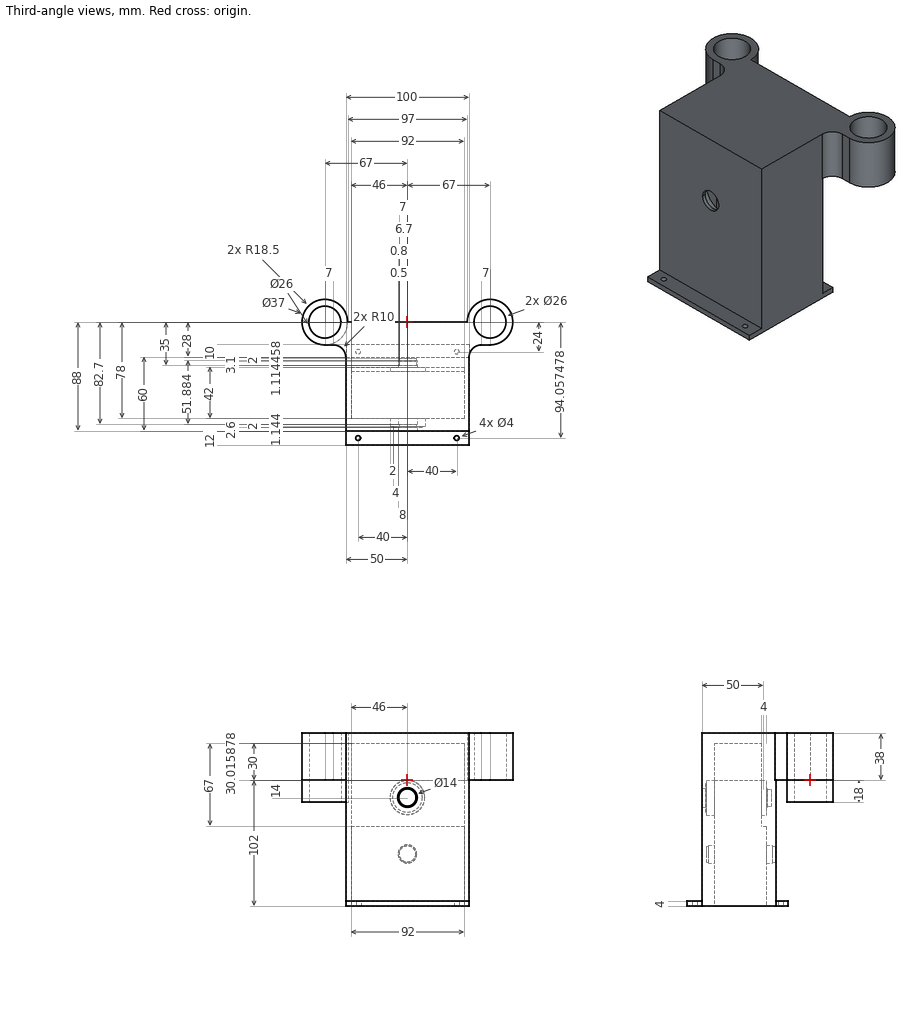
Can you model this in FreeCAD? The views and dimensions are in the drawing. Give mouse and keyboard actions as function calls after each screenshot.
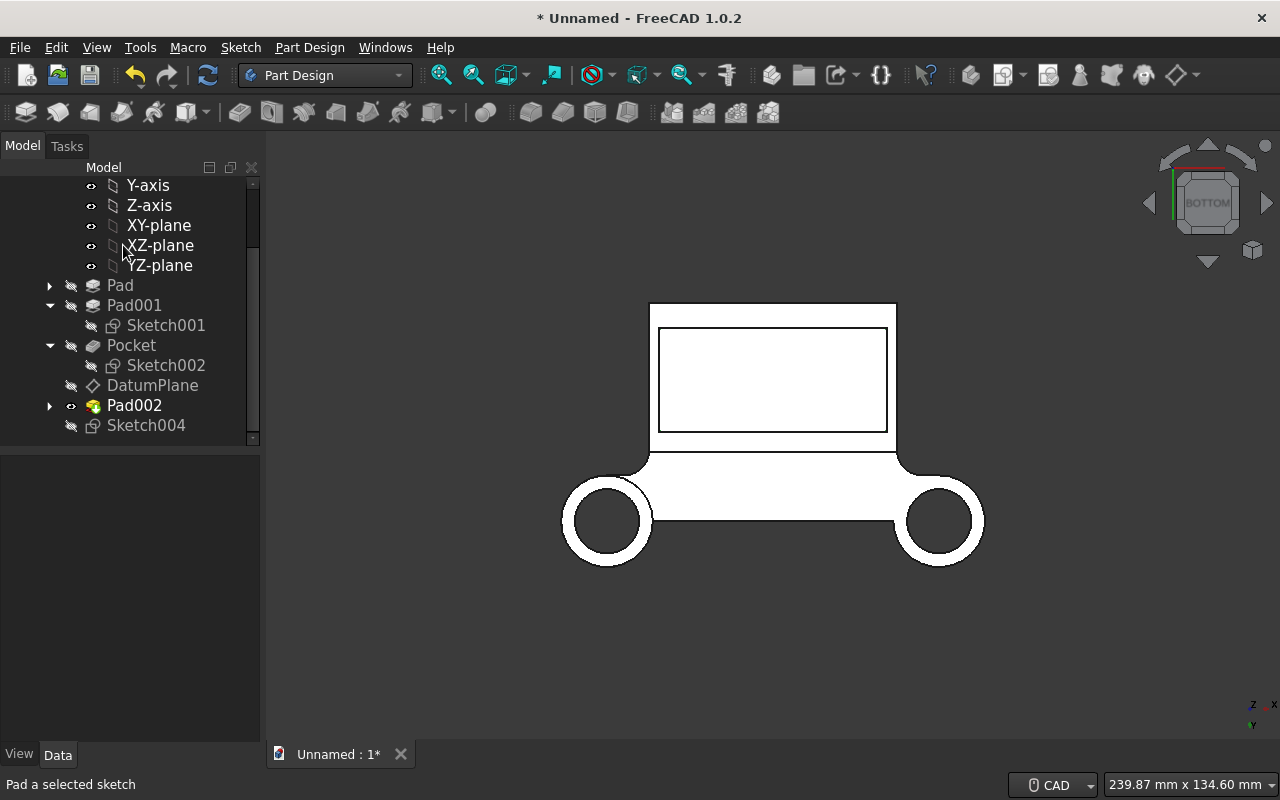
click(240, 112)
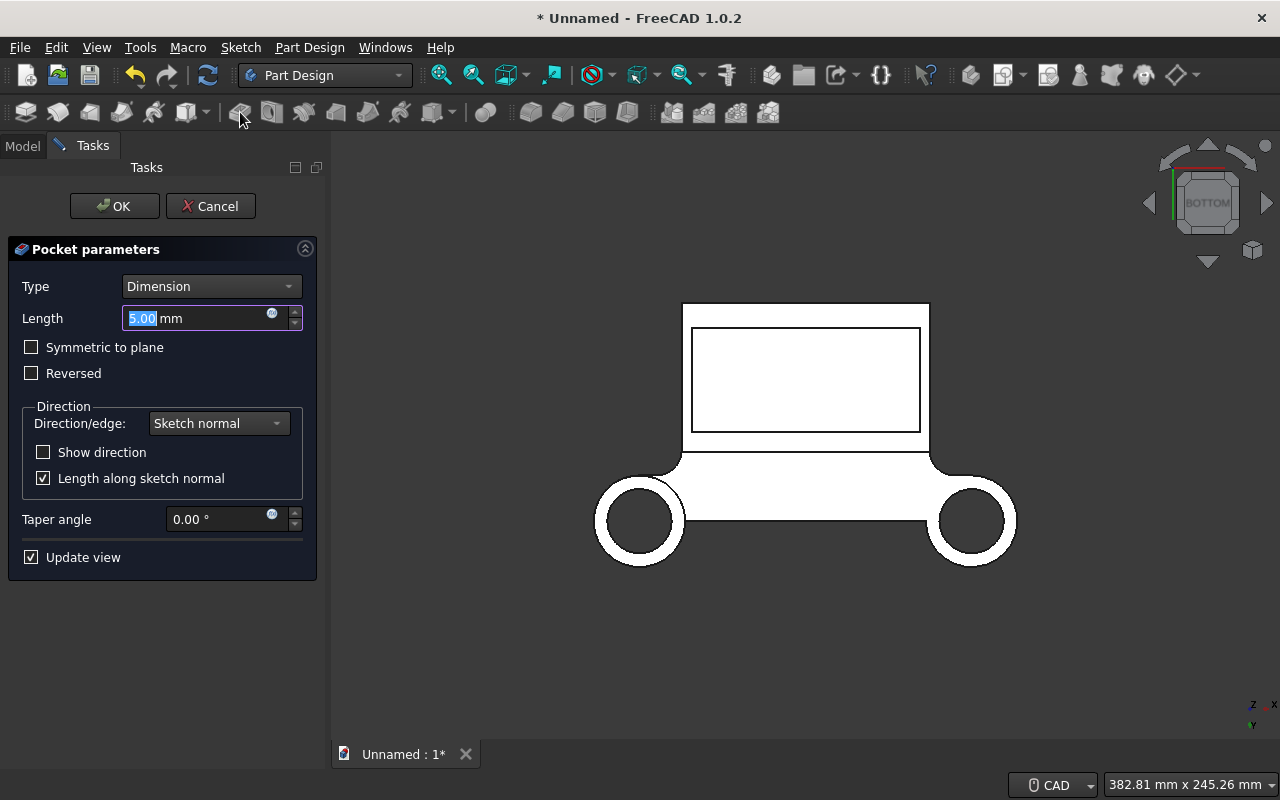
text(30)
key(Tab)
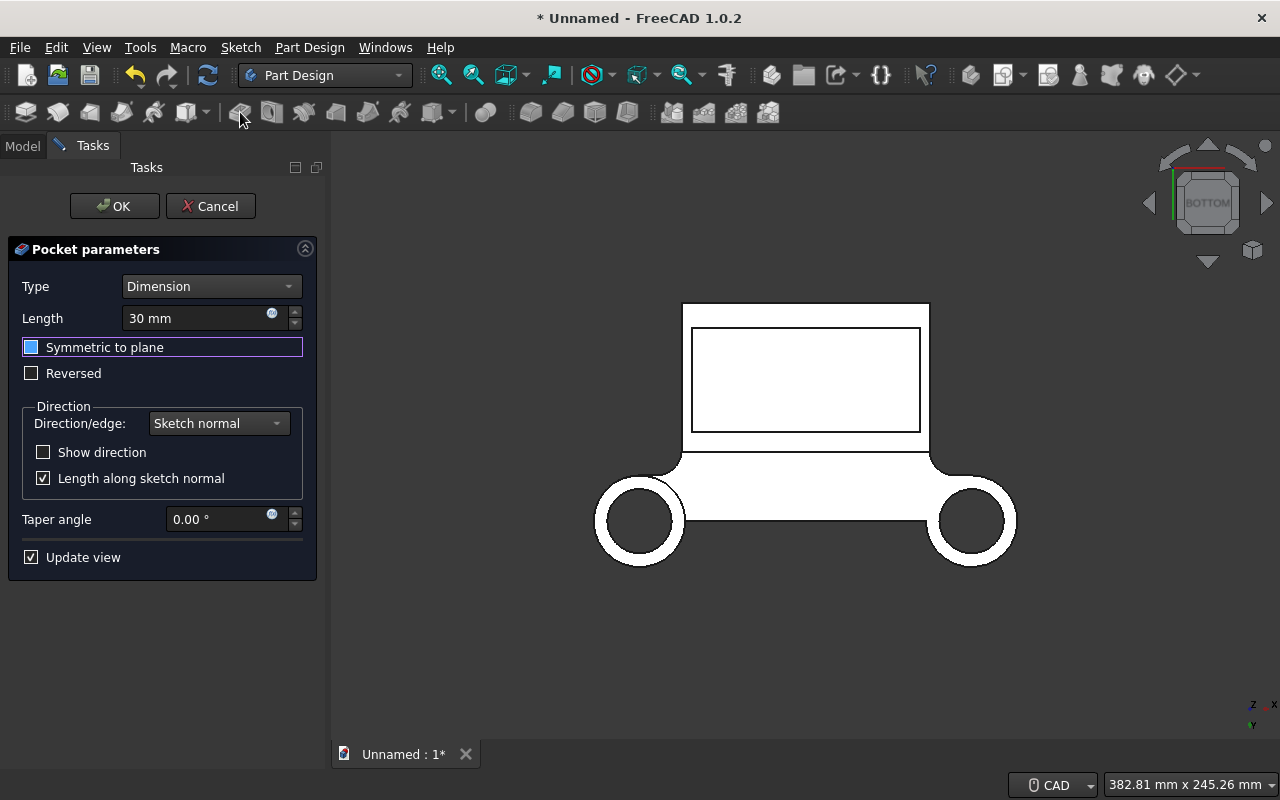
click(115, 206)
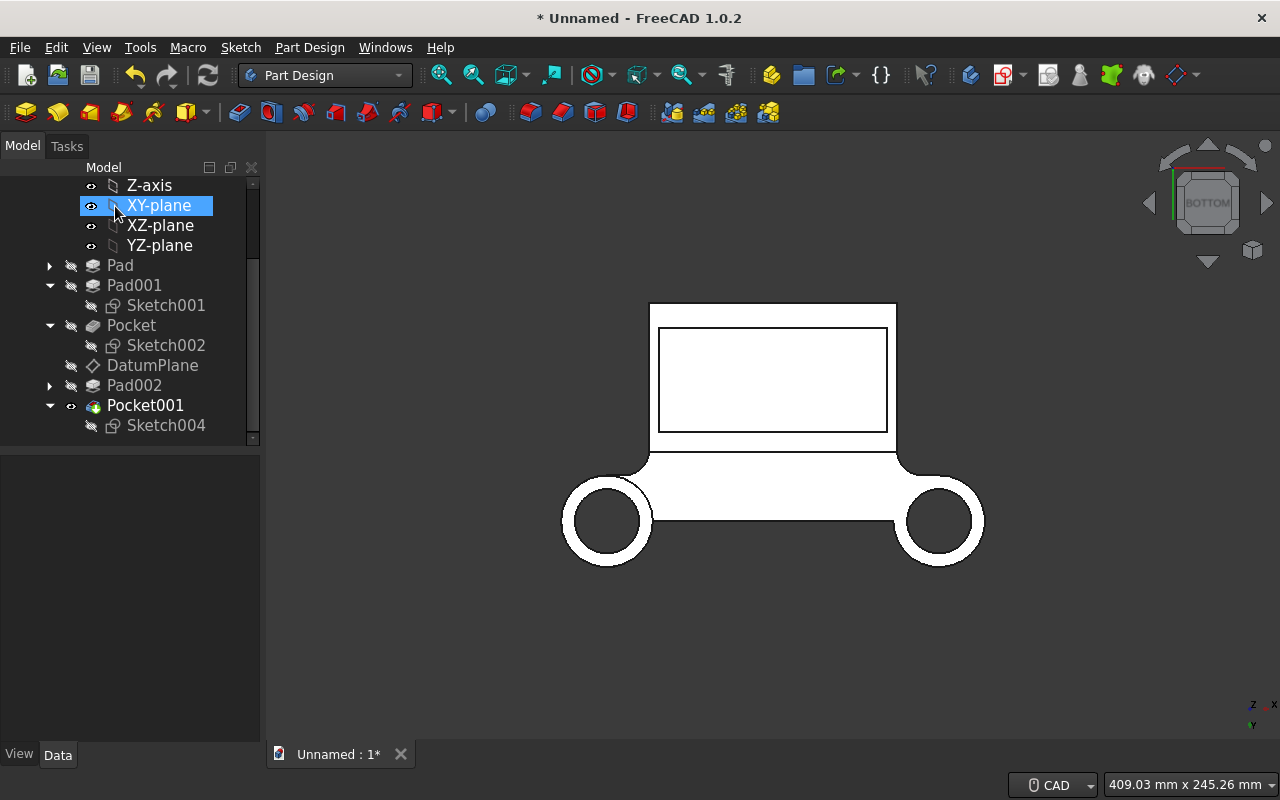
click(442, 76)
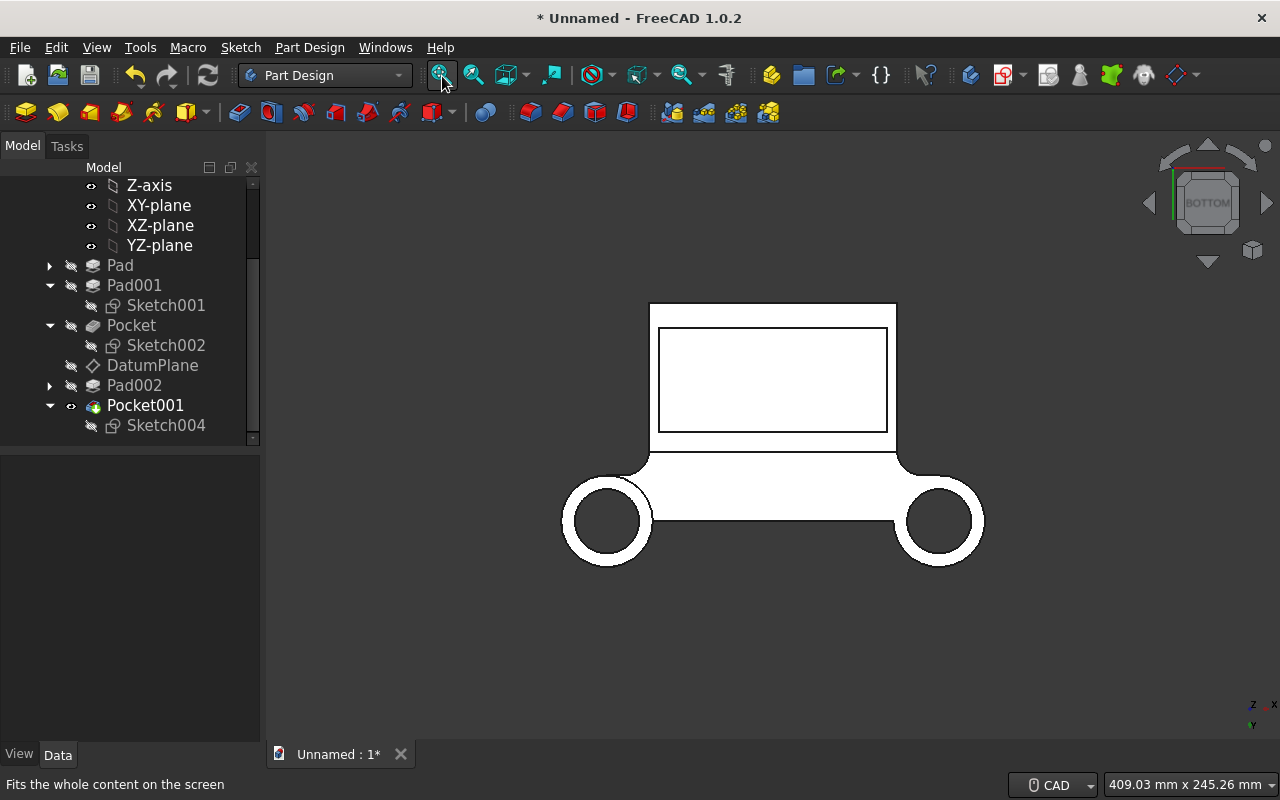
key(0)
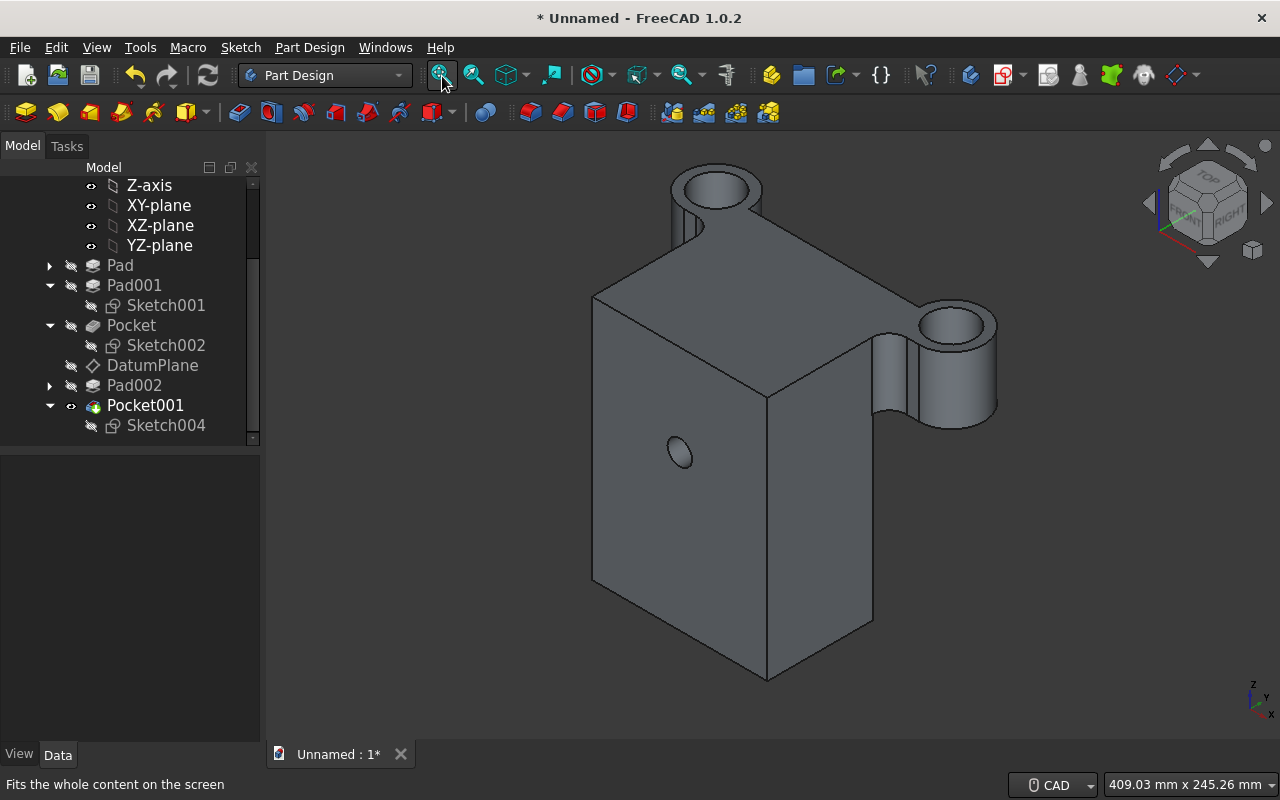
key(1)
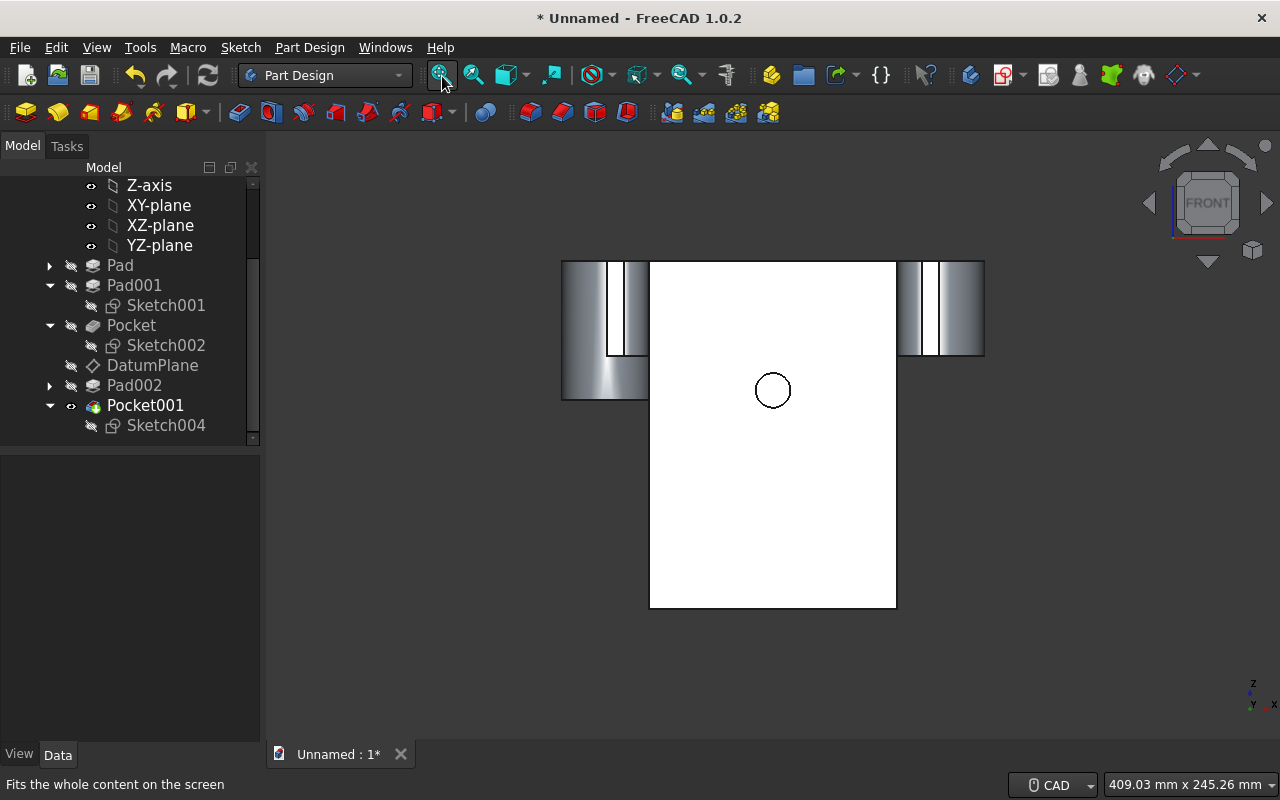
click(773, 397)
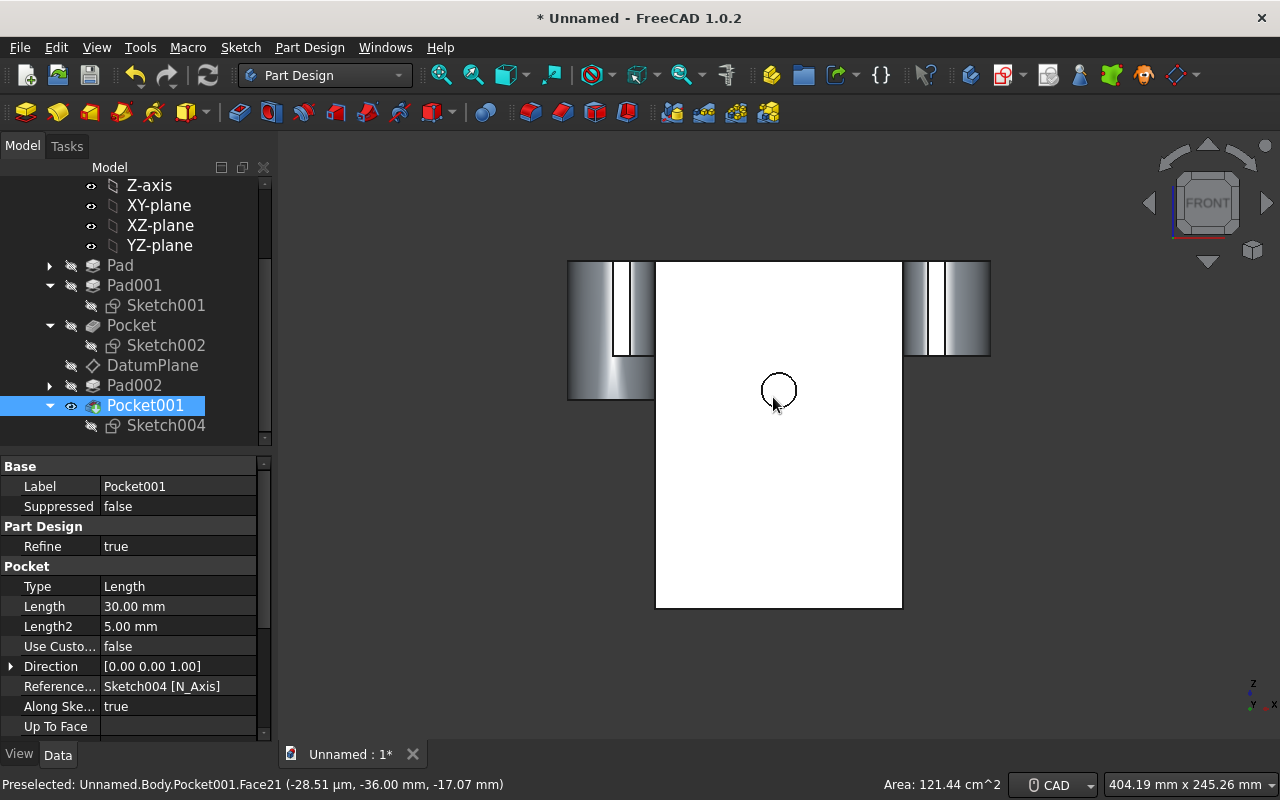
click(1004, 76)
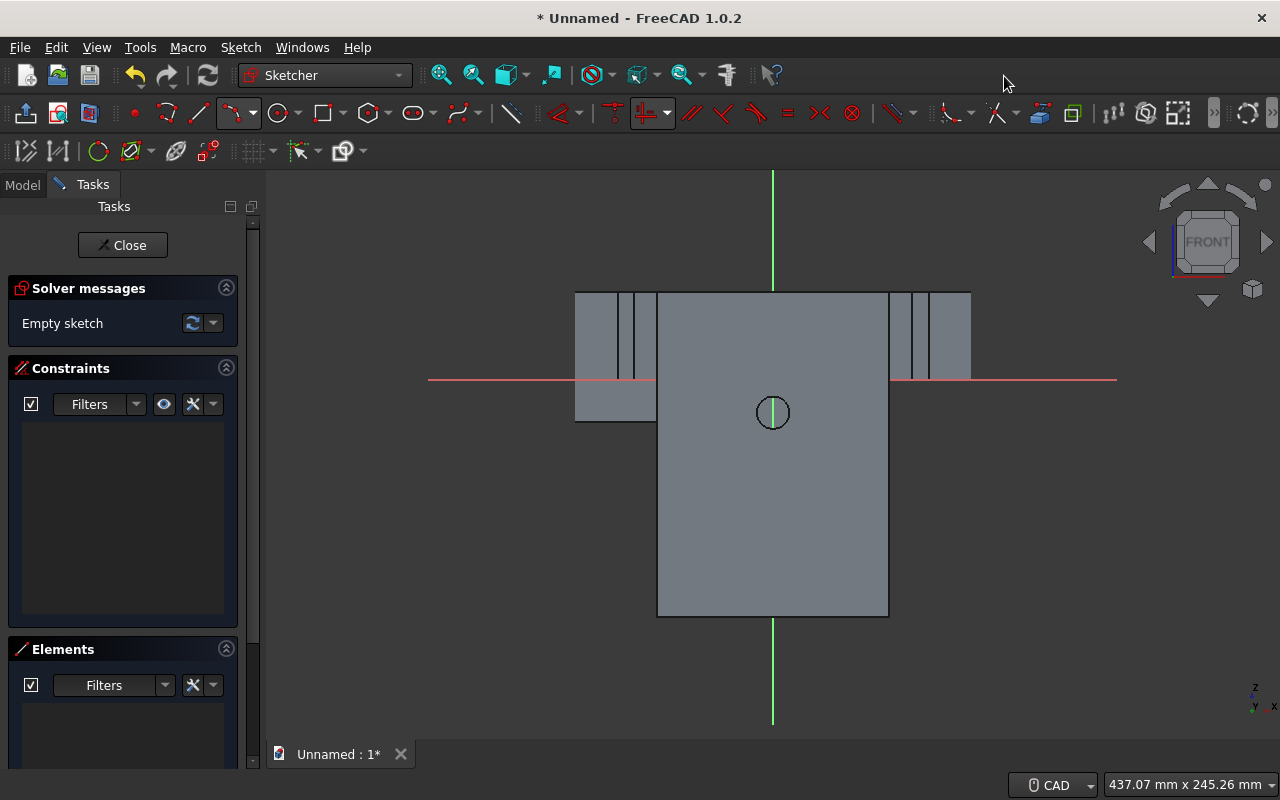
scroll(829, 334, up, 4)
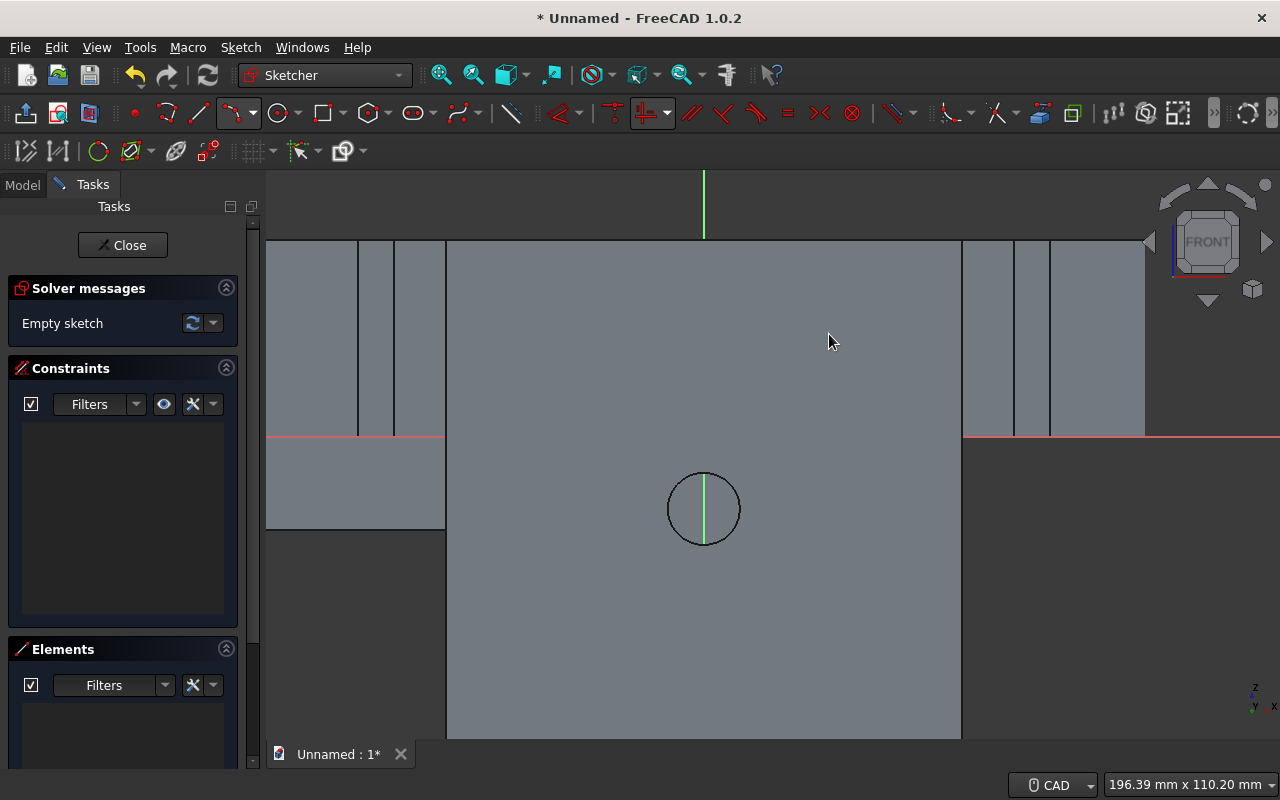
key(g)
key(r)